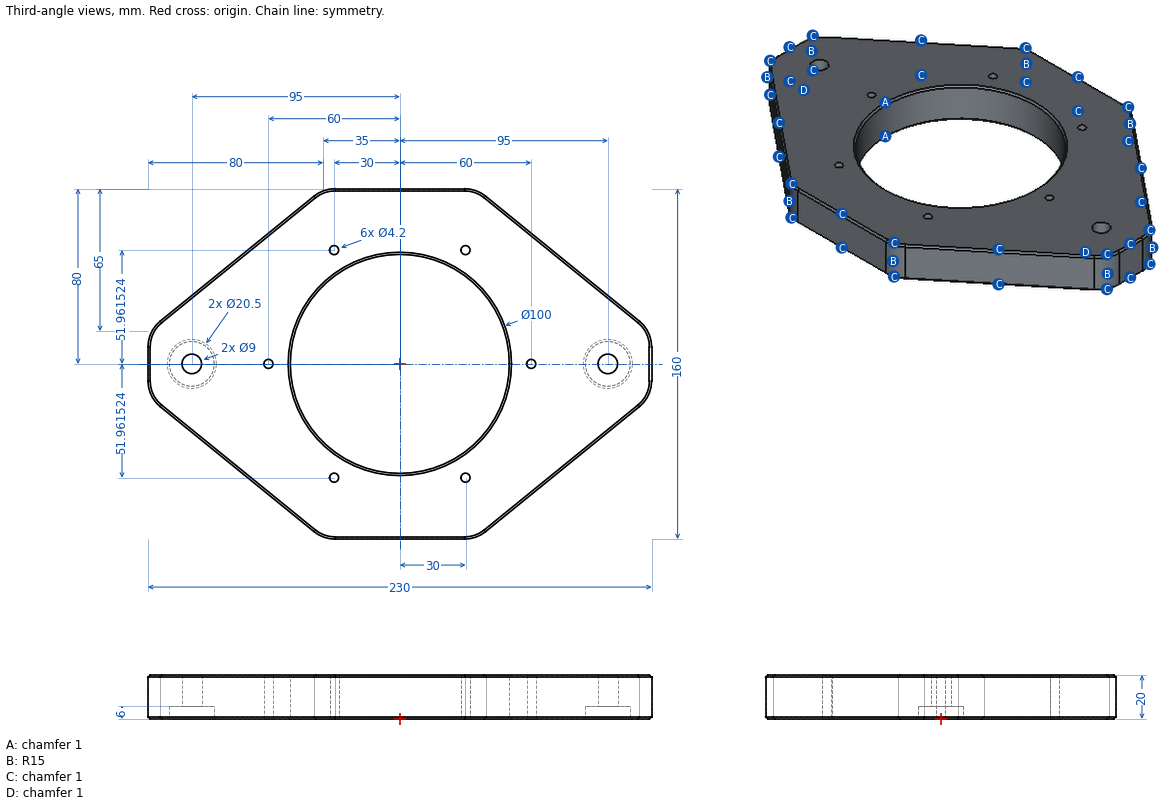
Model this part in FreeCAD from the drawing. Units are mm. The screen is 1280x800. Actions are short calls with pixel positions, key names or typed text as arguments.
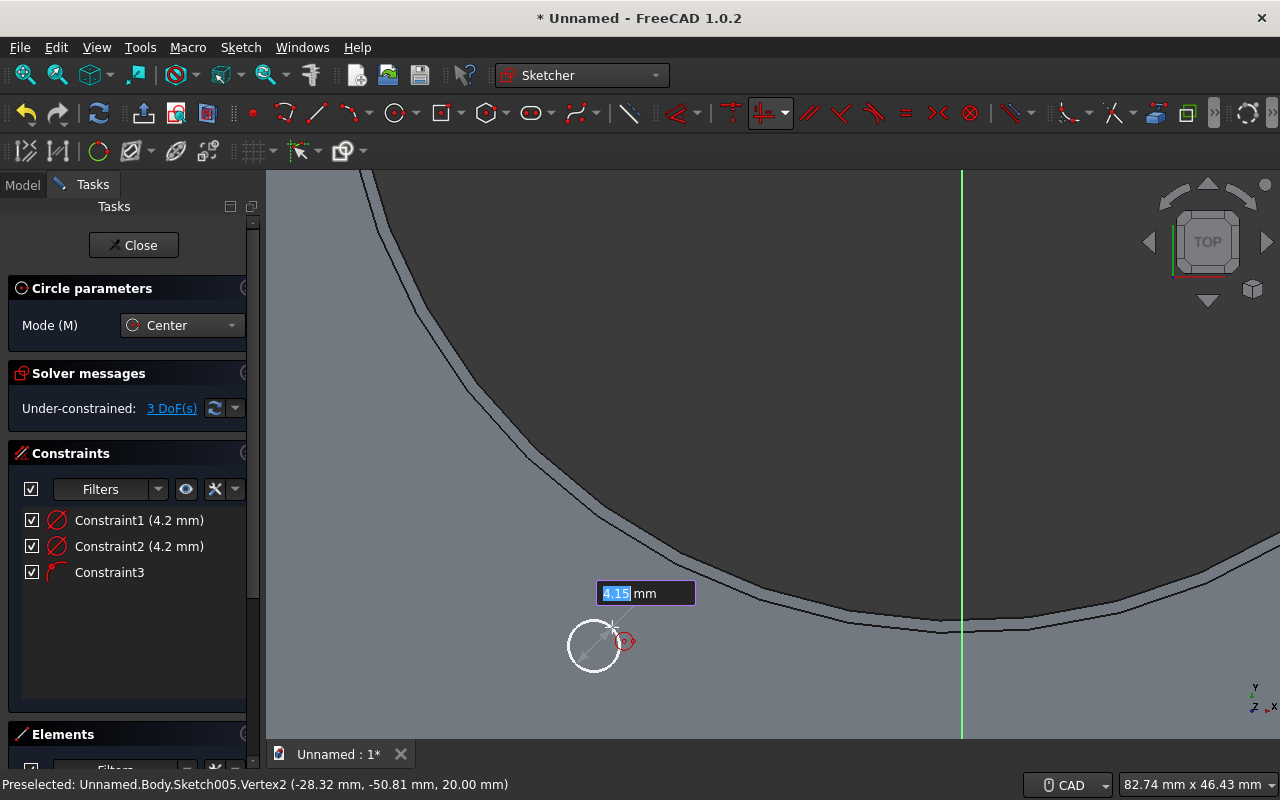
text(4.2)
key(Return)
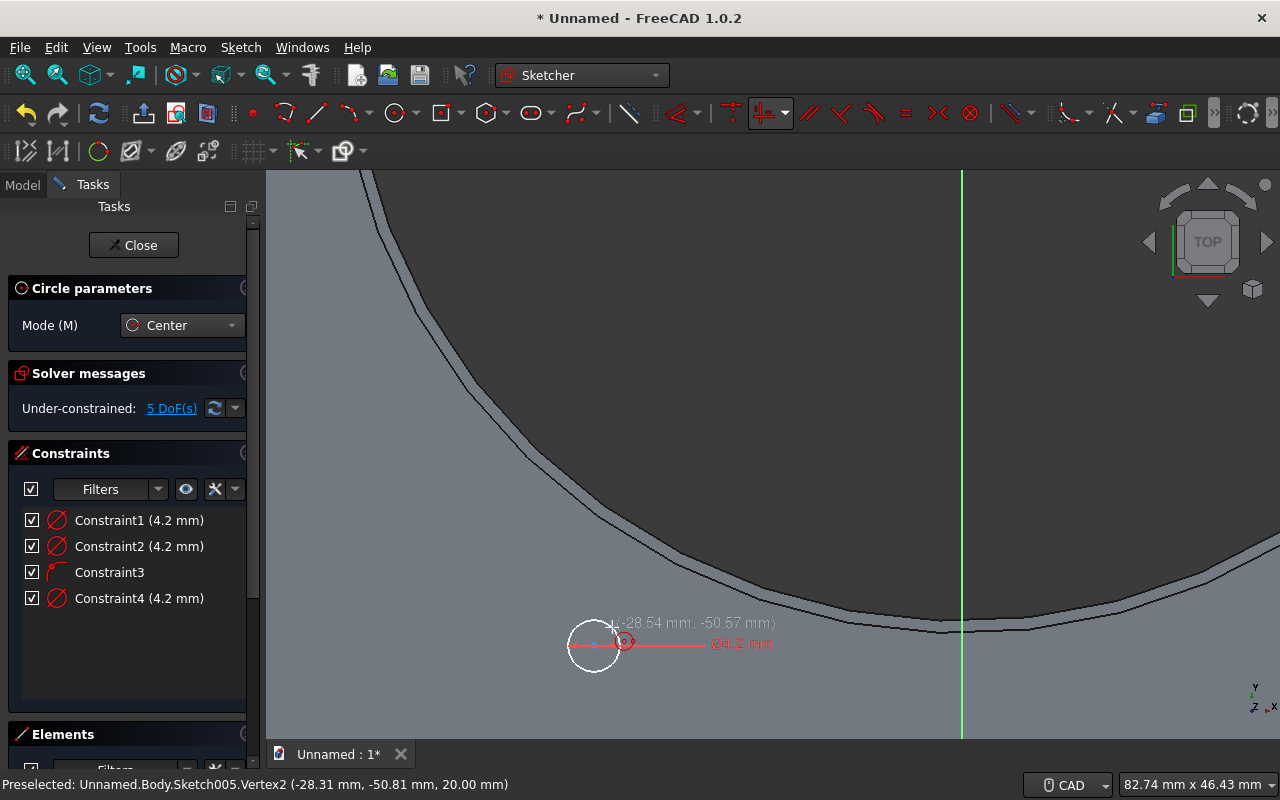
scroll(594, 647, down, 6)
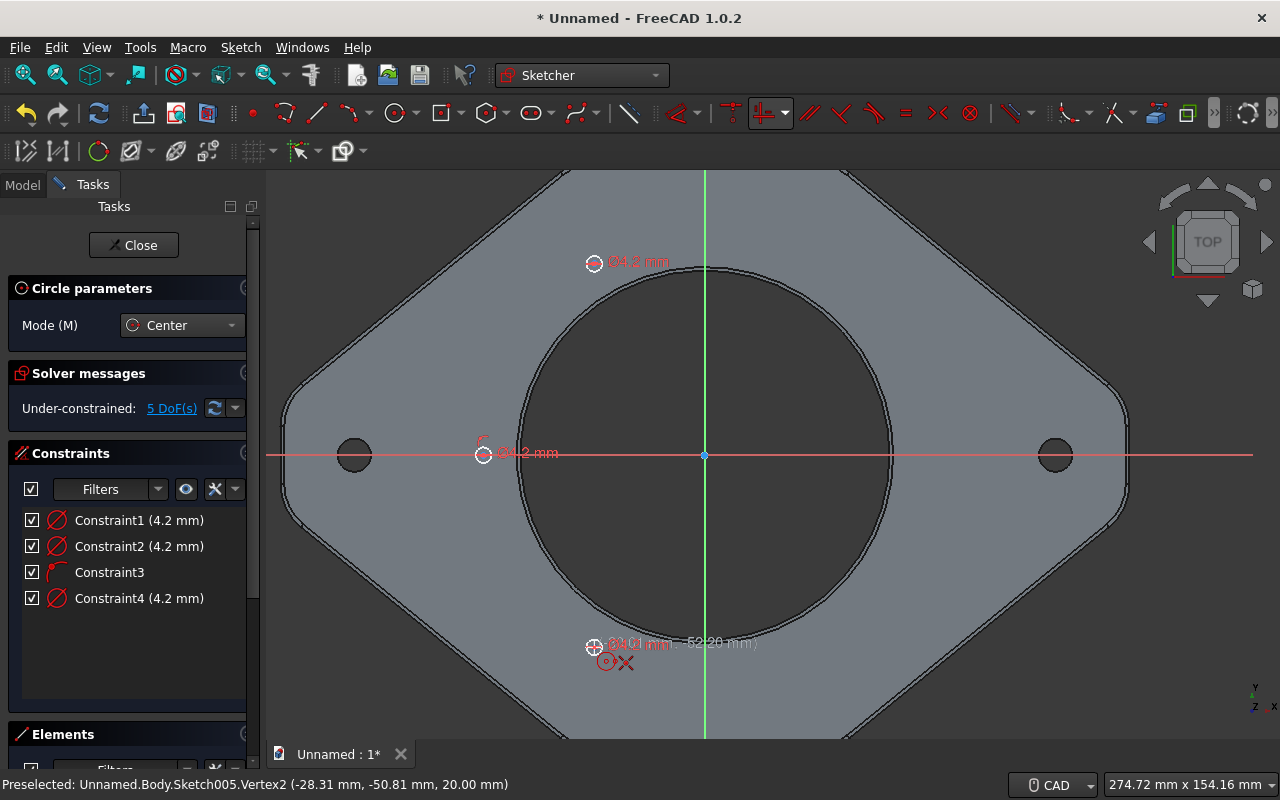
scroll(816, 647, up, 6)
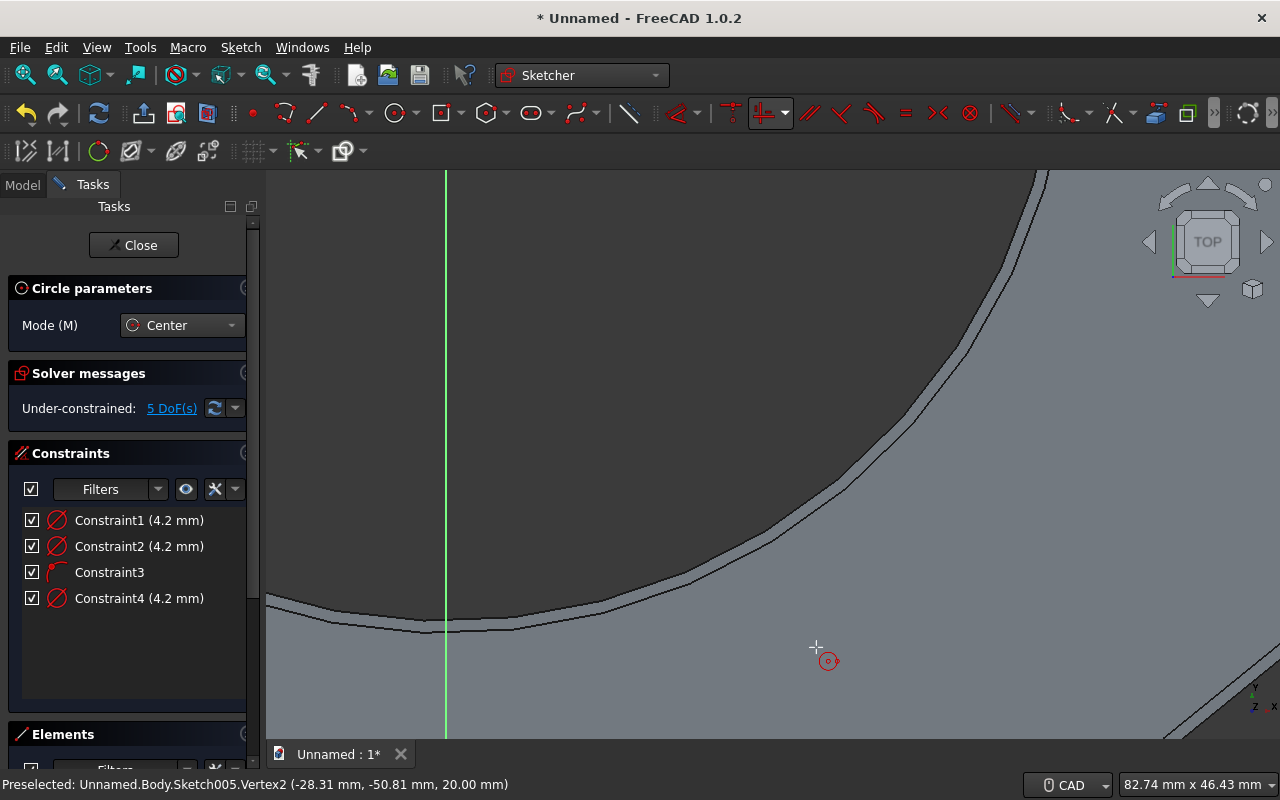
click(814, 645)
move(832, 627)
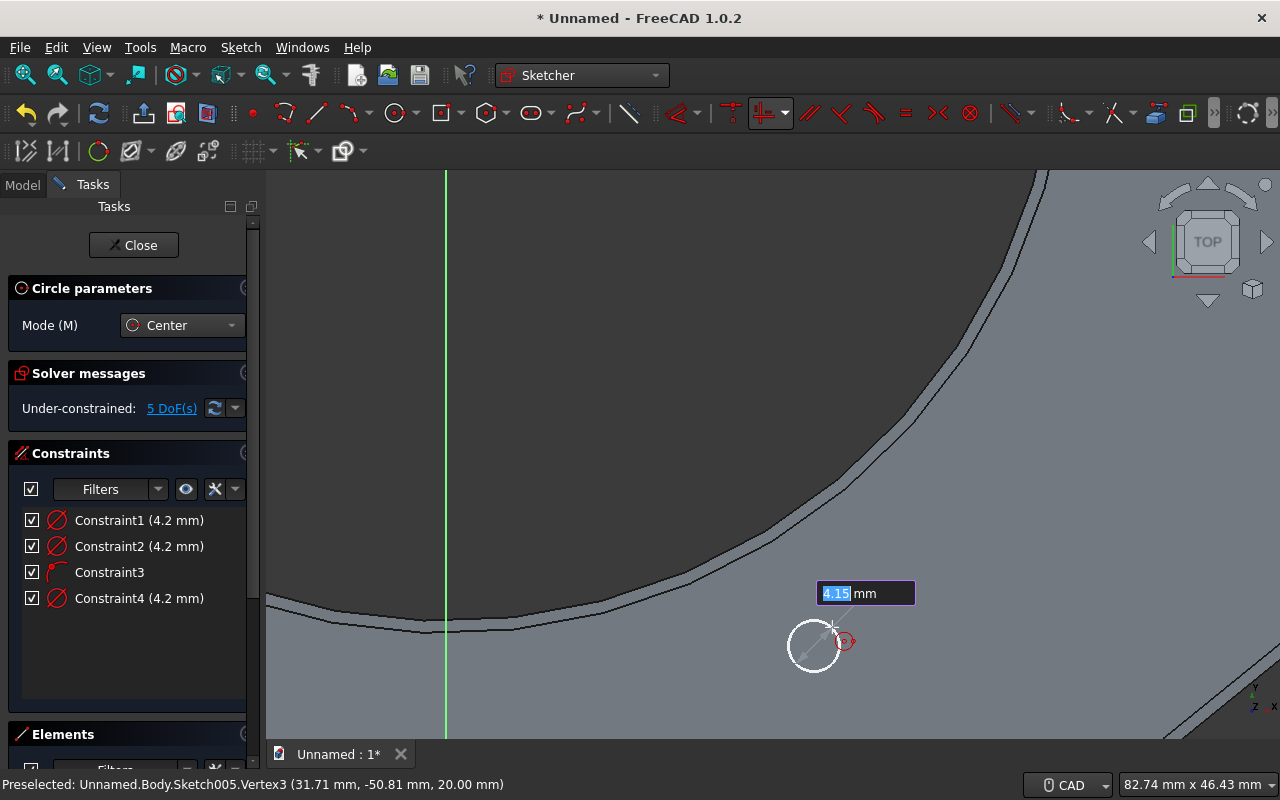
text(4.2)
key(Return)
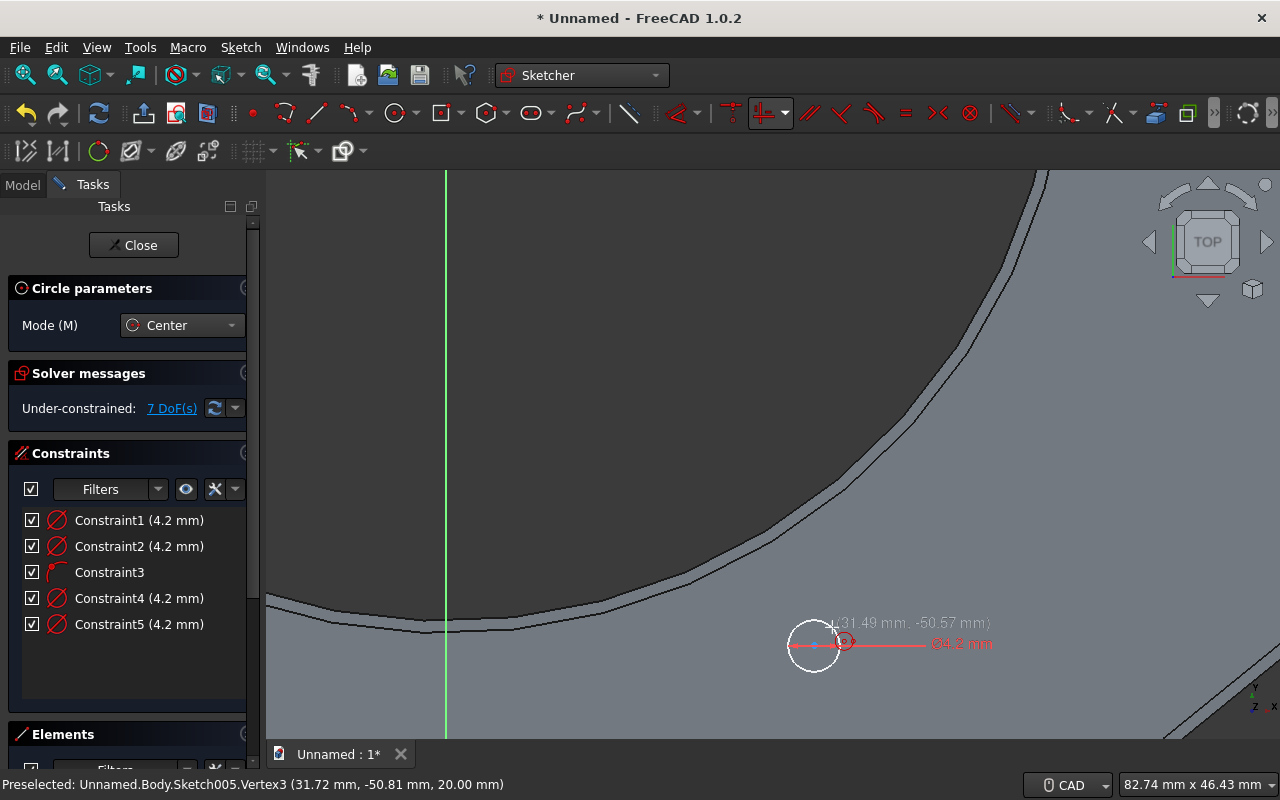
scroll(816, 647, down, 6)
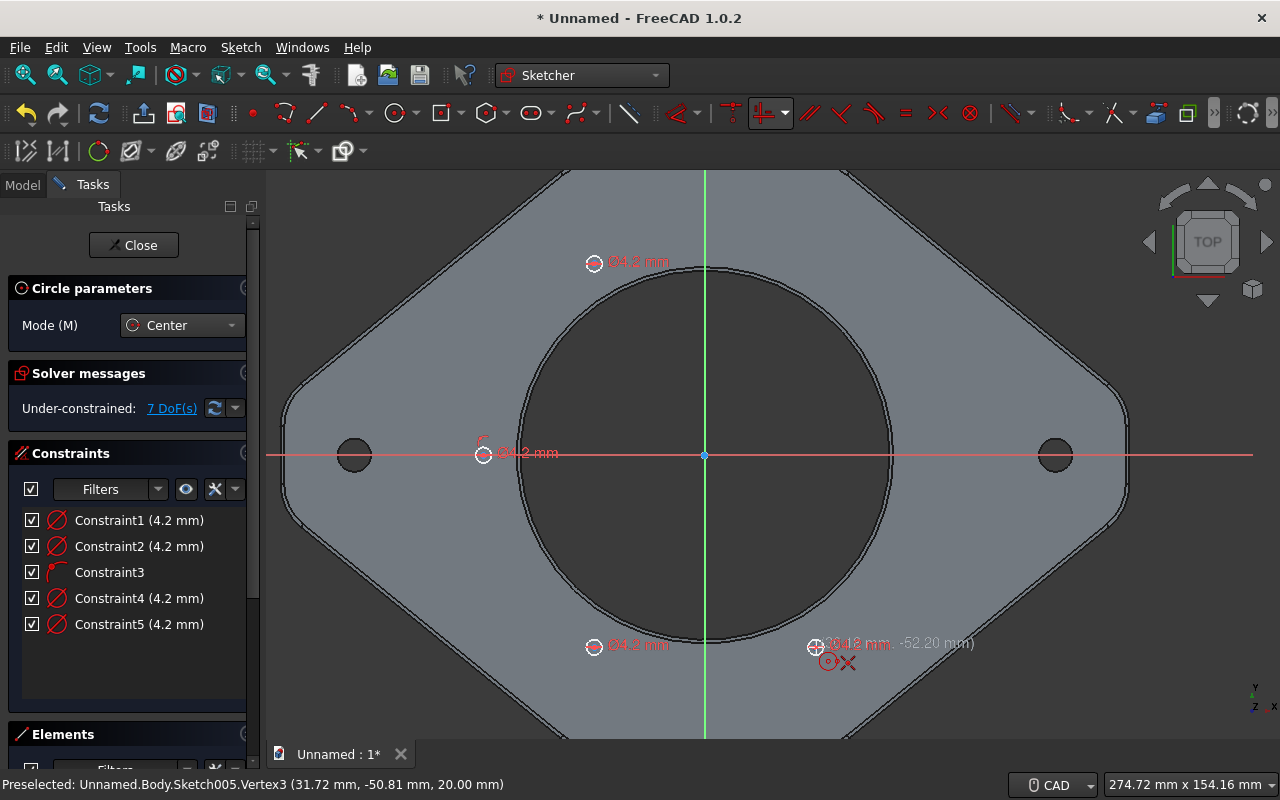
scroll(926, 455, up, 6)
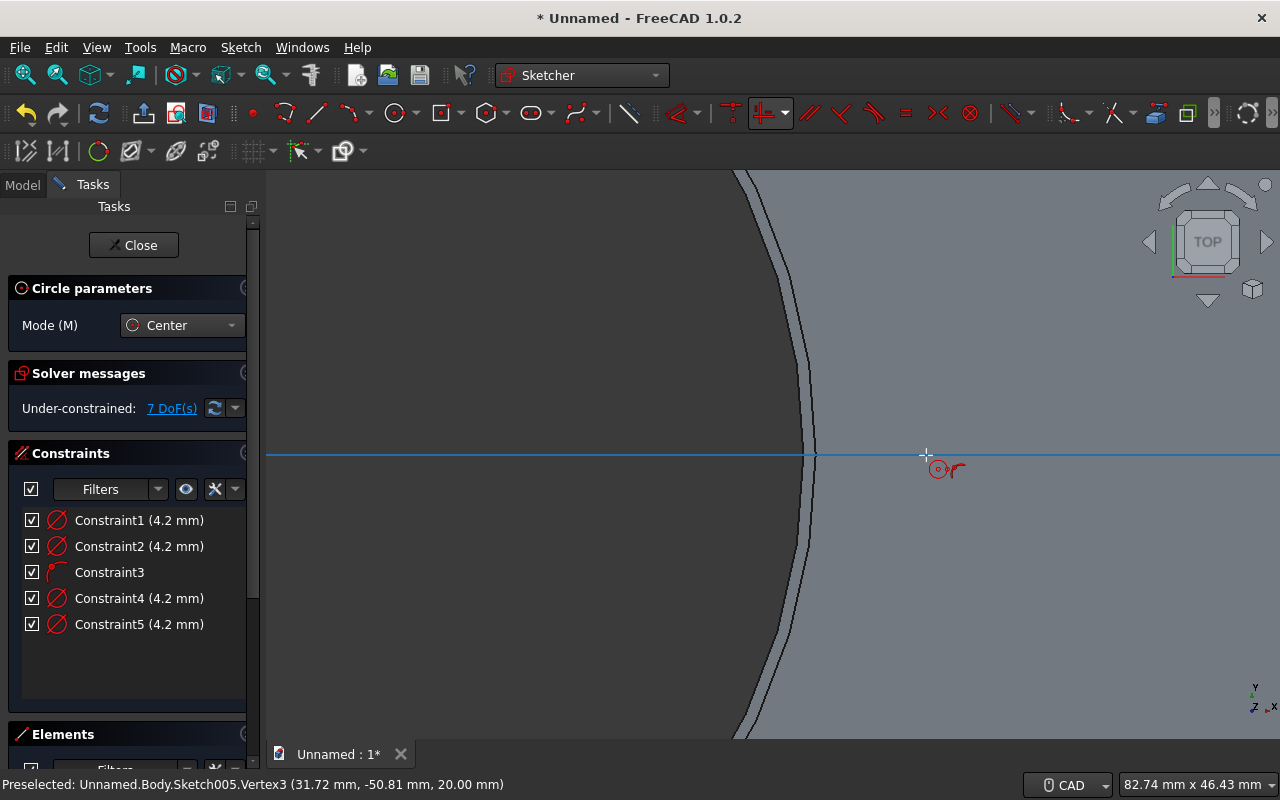
click(926, 454)
move(944, 436)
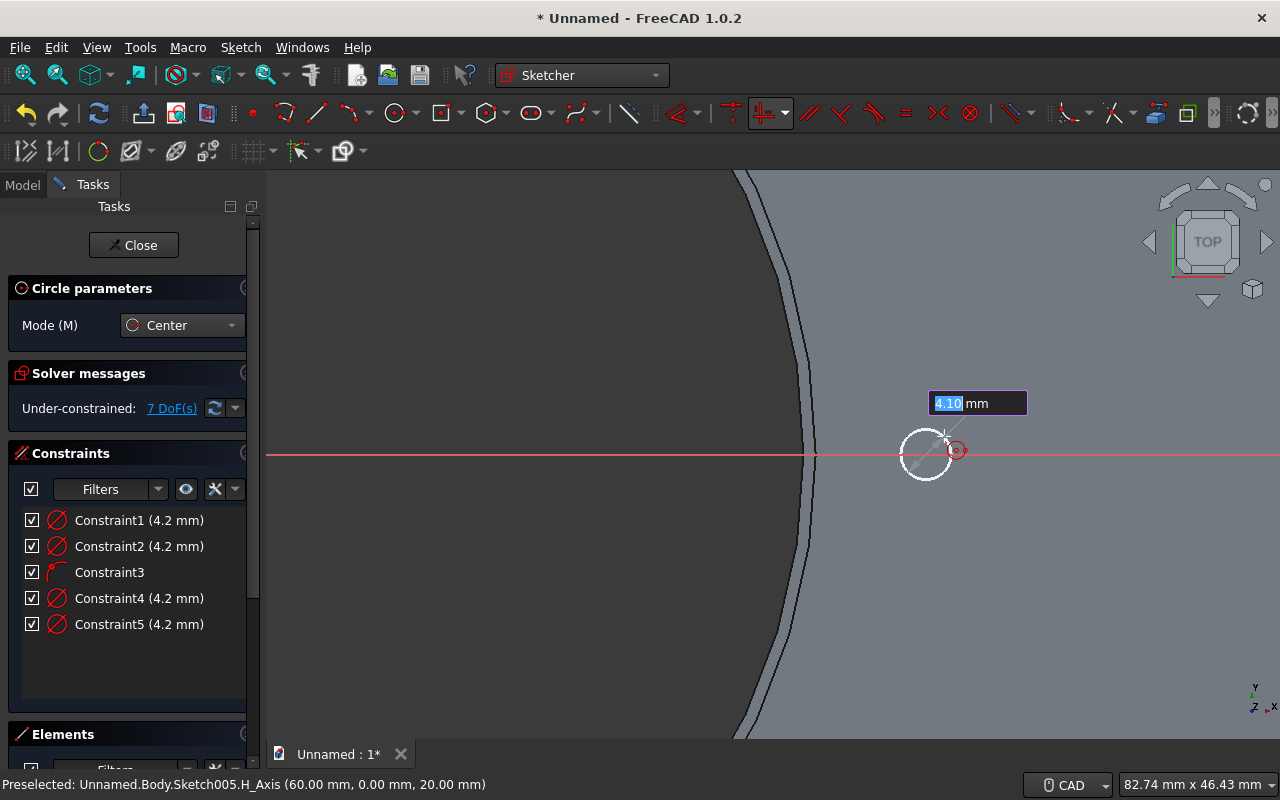
text(4.2)
key(Return)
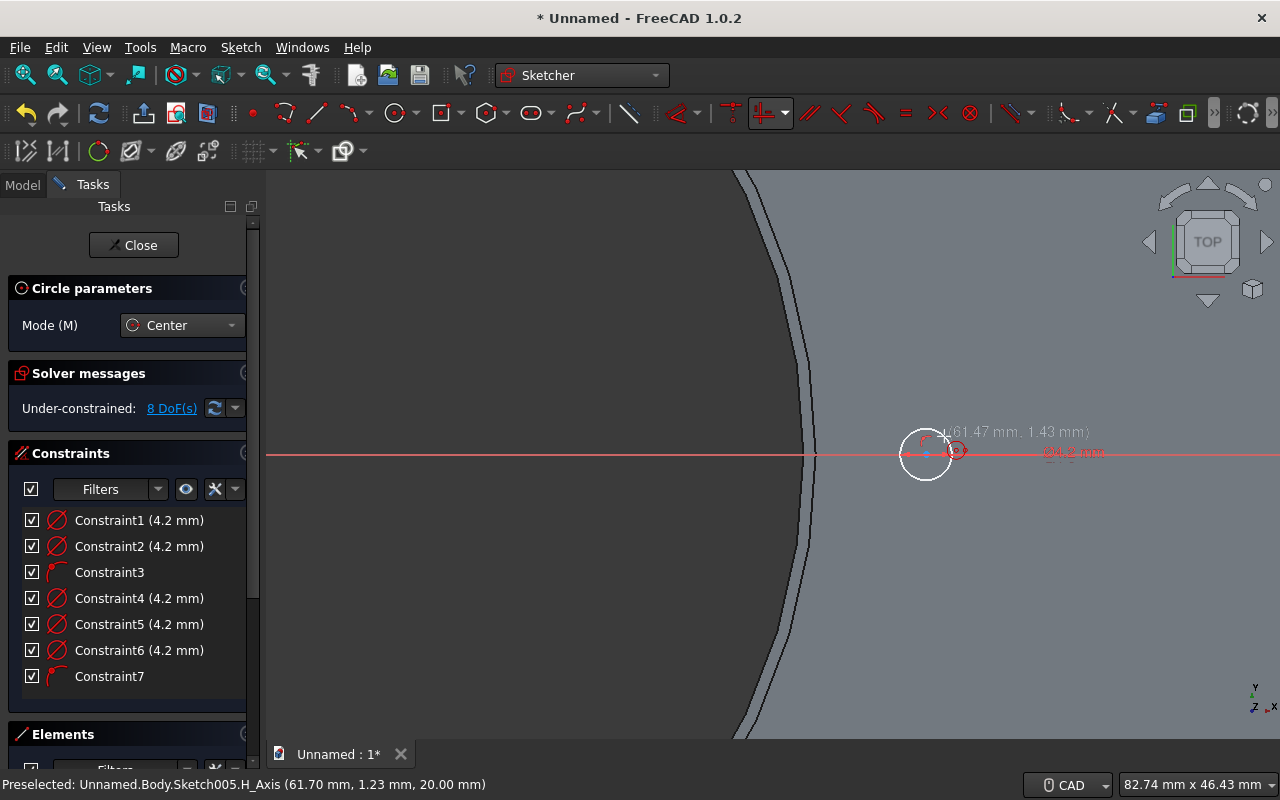
scroll(926, 455, down, 6)